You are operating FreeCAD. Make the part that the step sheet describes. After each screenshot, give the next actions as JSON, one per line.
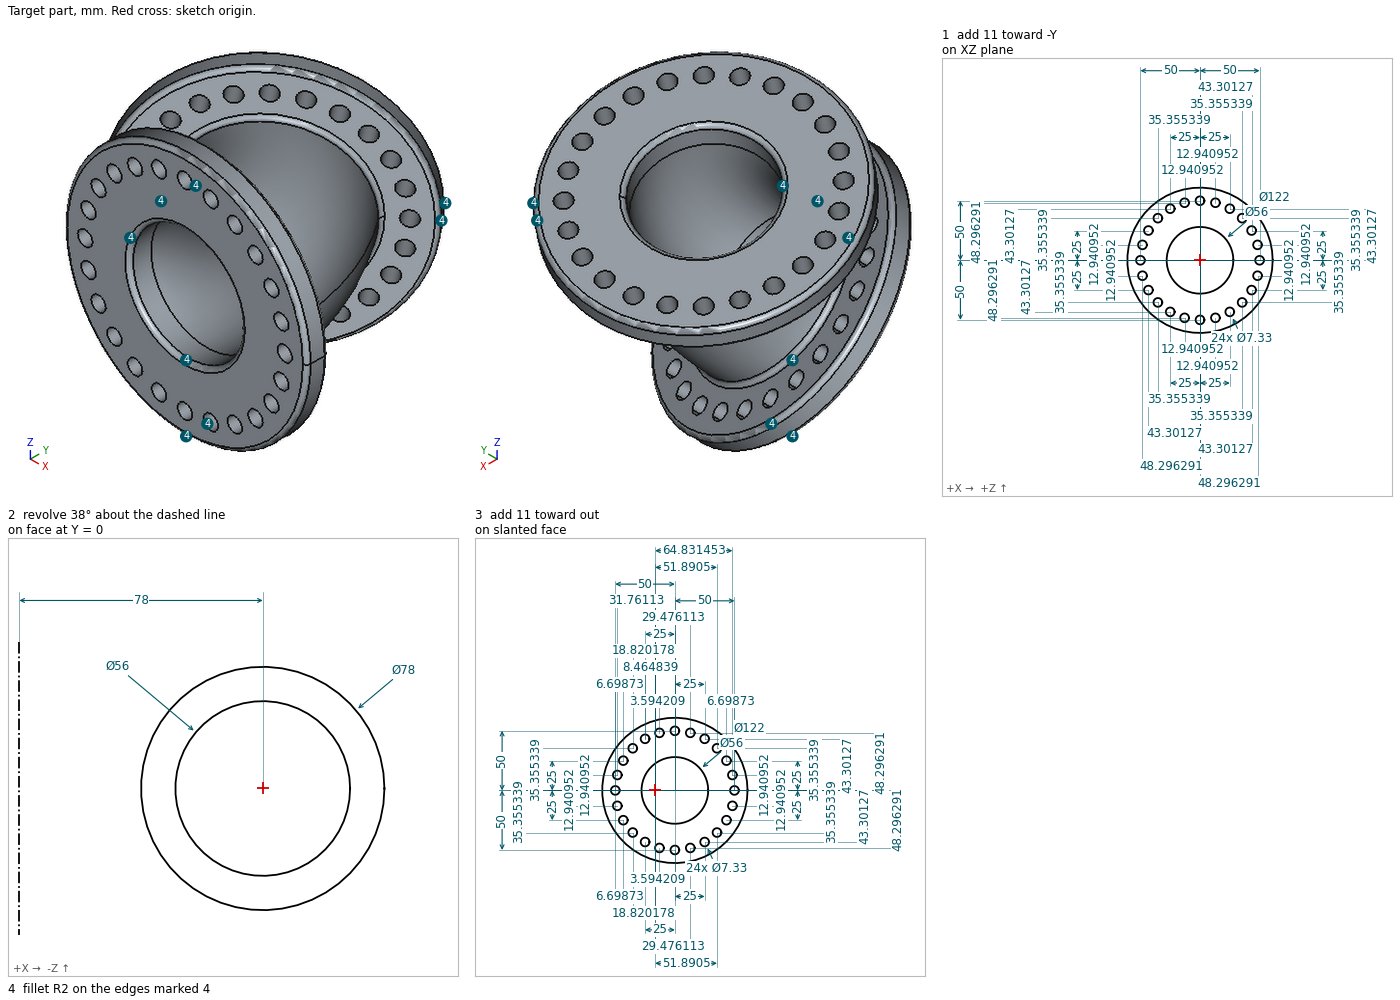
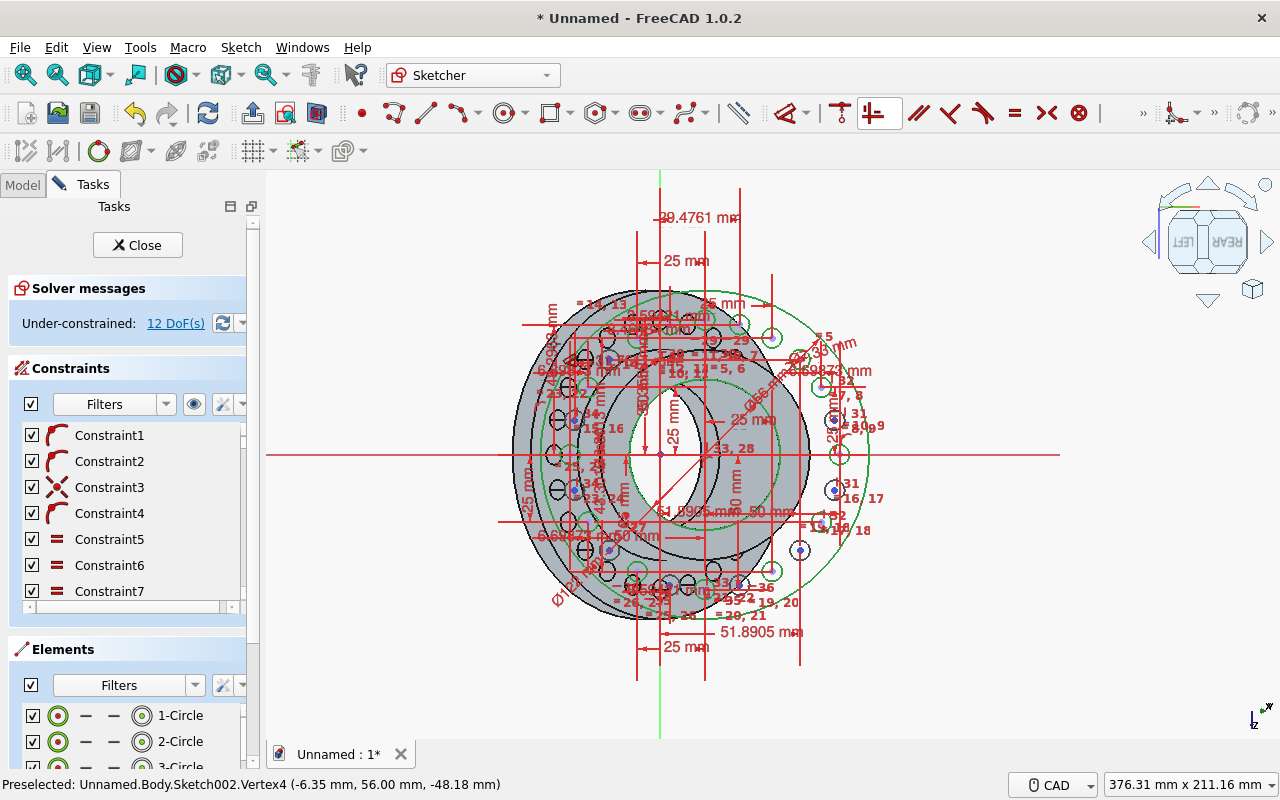
{"action": "left_click", "coordinate": [835, 420]}
{"action": "left_click", "coordinate": [809, 489]}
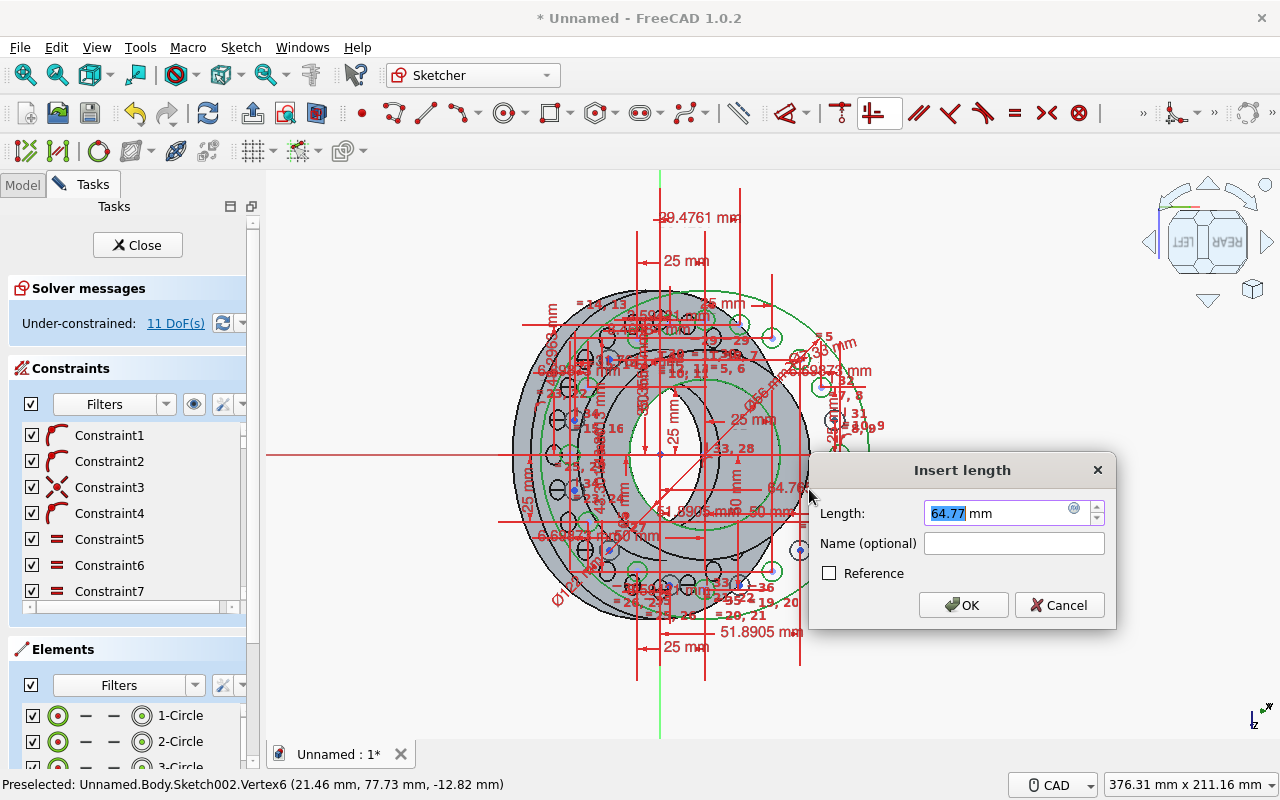
{"action": "type", "text": "64.831453"}
{"action": "key", "text": "Return"}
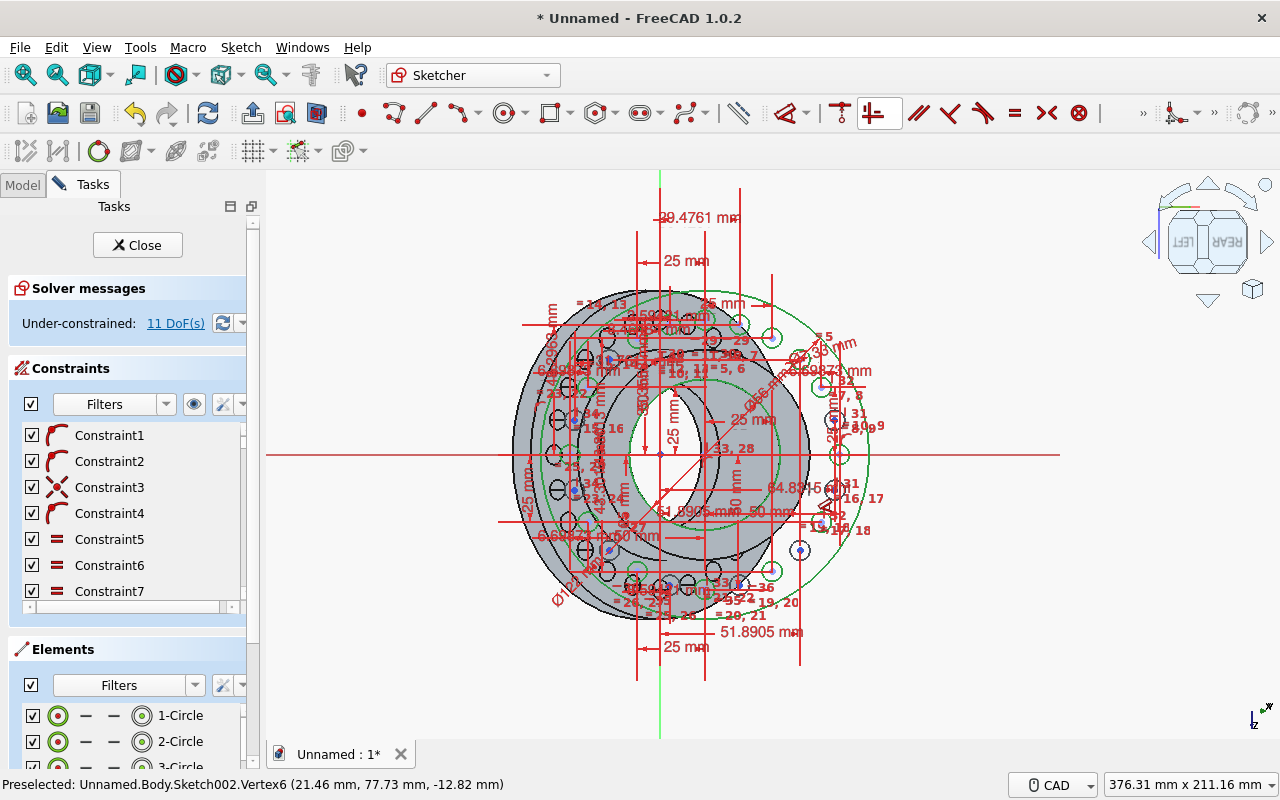
{"action": "left_click", "coordinate": [835, 420]}
{"action": "left_click", "coordinate": [917, 438]}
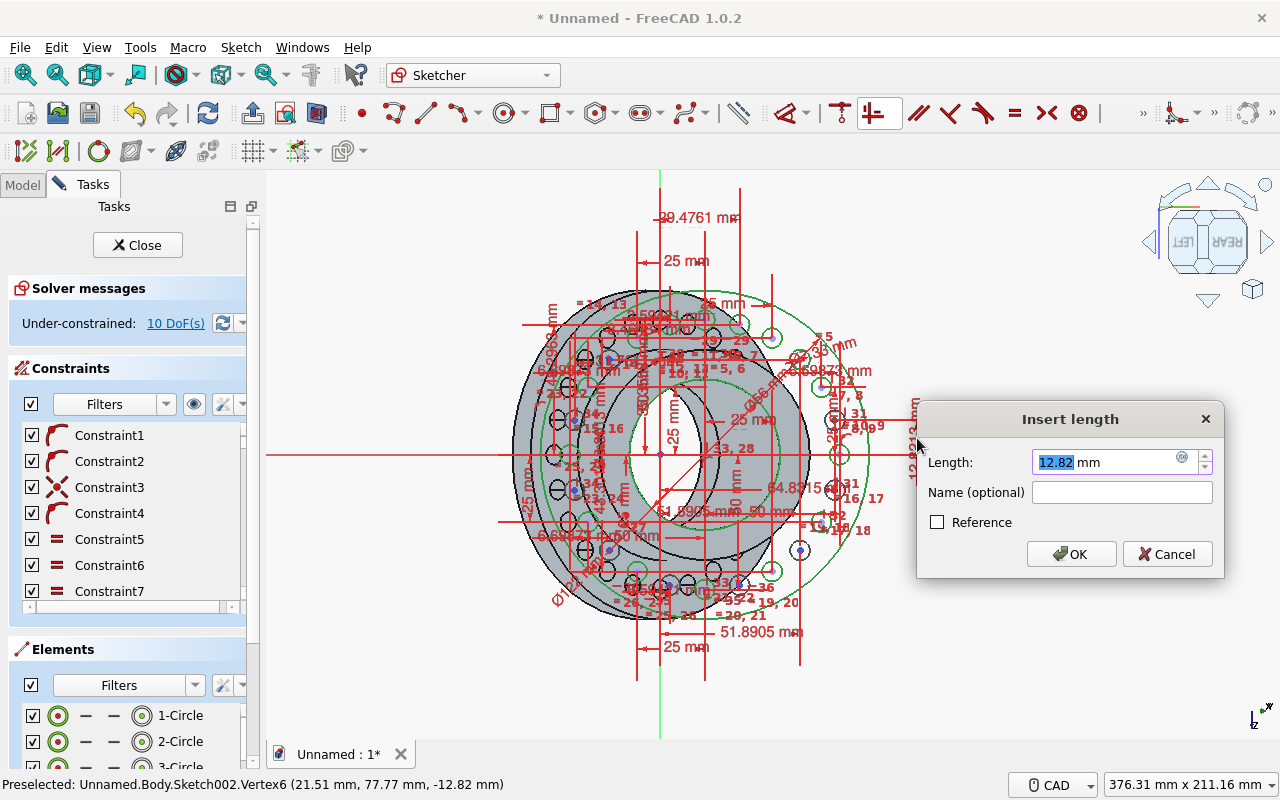
{"action": "type", "text": "12.940952"}
{"action": "key", "text": "Return"}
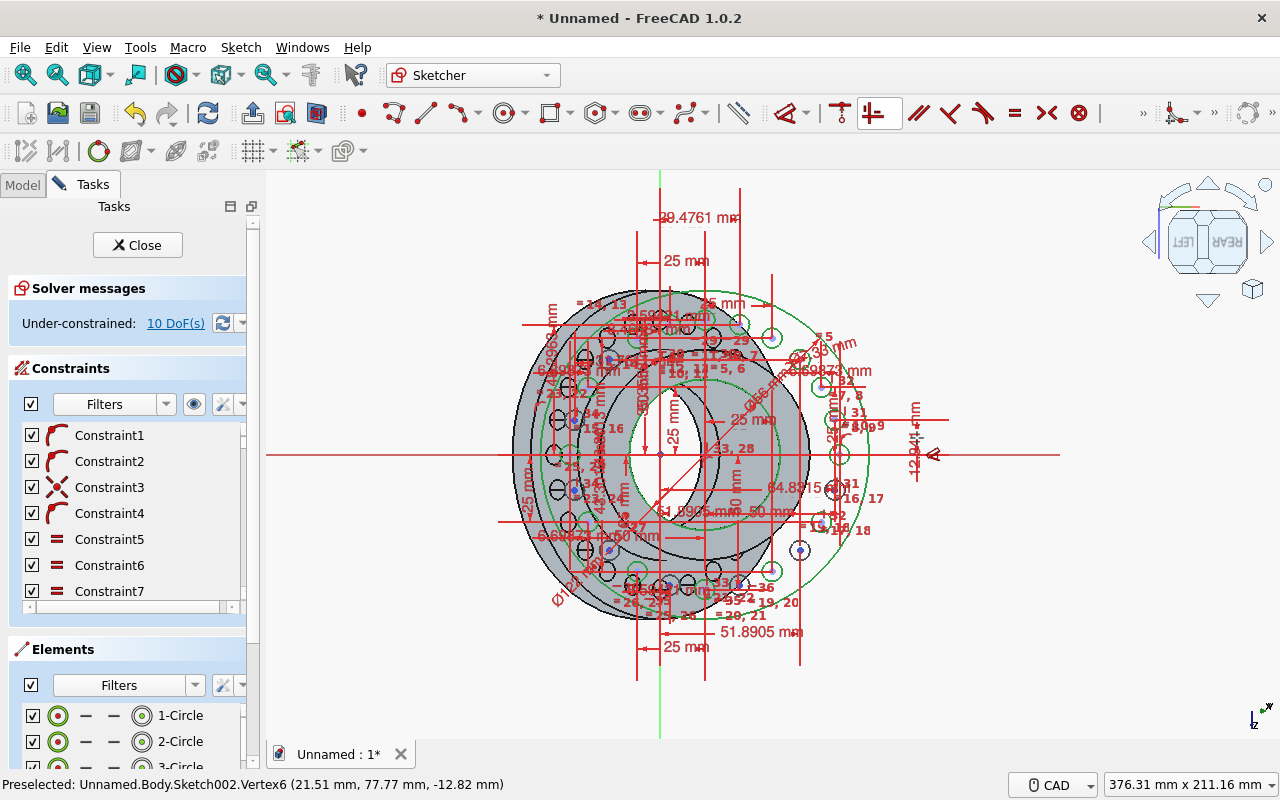
{"action": "left_click", "coordinate": [610, 360]}
{"action": "left_click", "coordinate": [623, 230]}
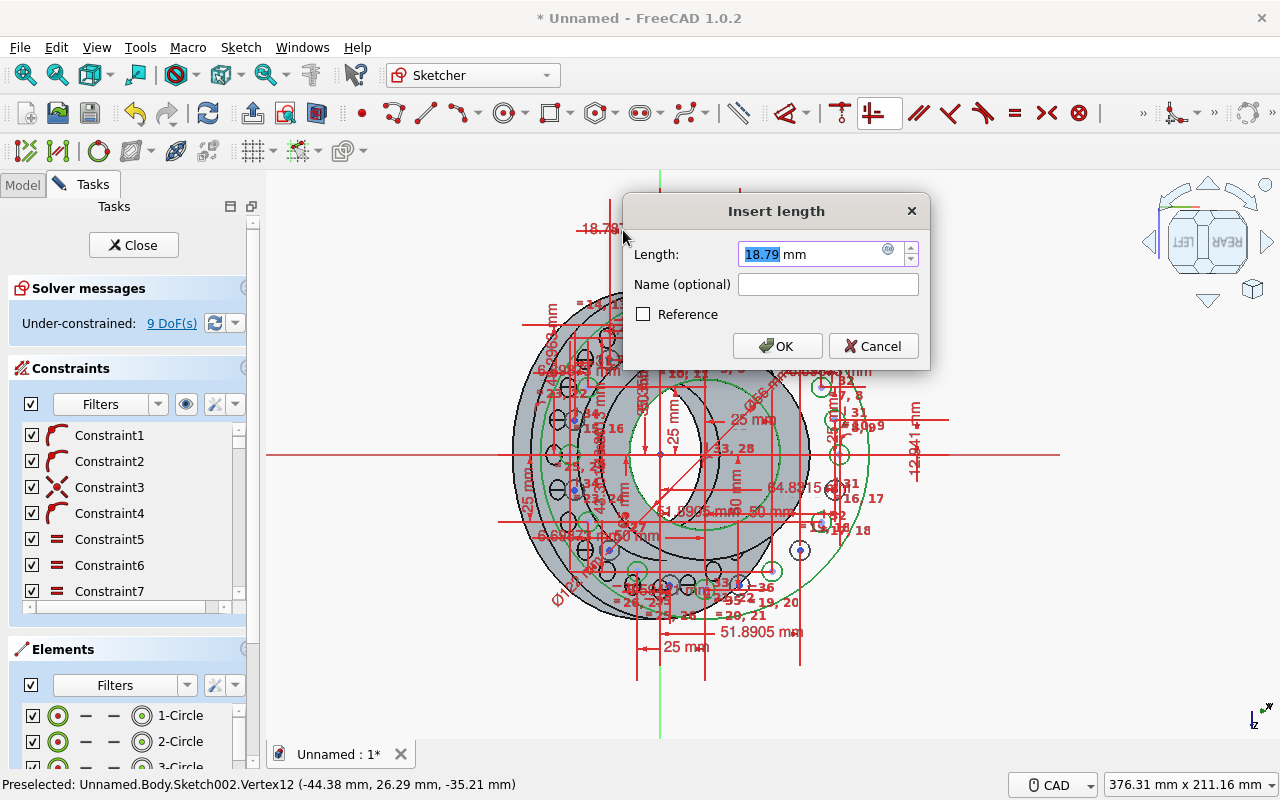
{"action": "type", "text": "18.820178"}
{"action": "key", "text": "Return"}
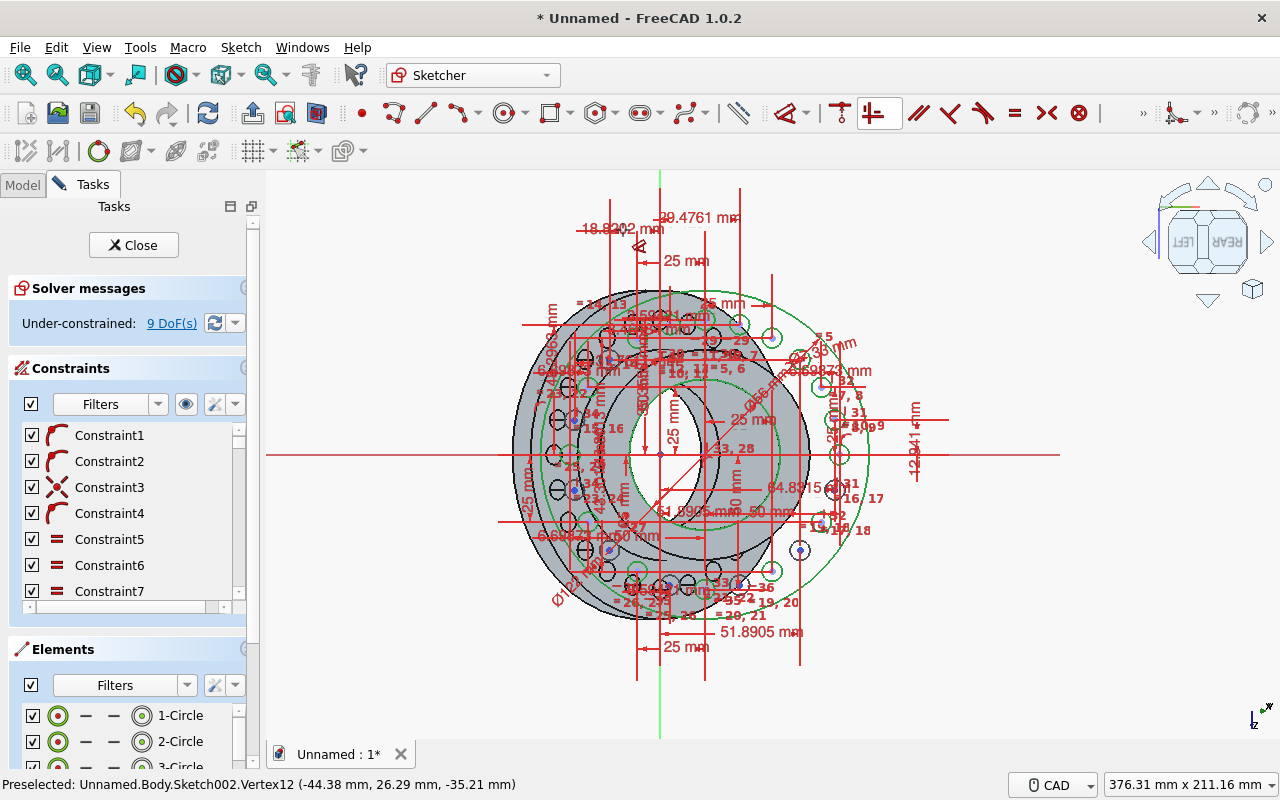
{"action": "left_click", "coordinate": [610, 360]}
{"action": "left_click", "coordinate": [528, 407]}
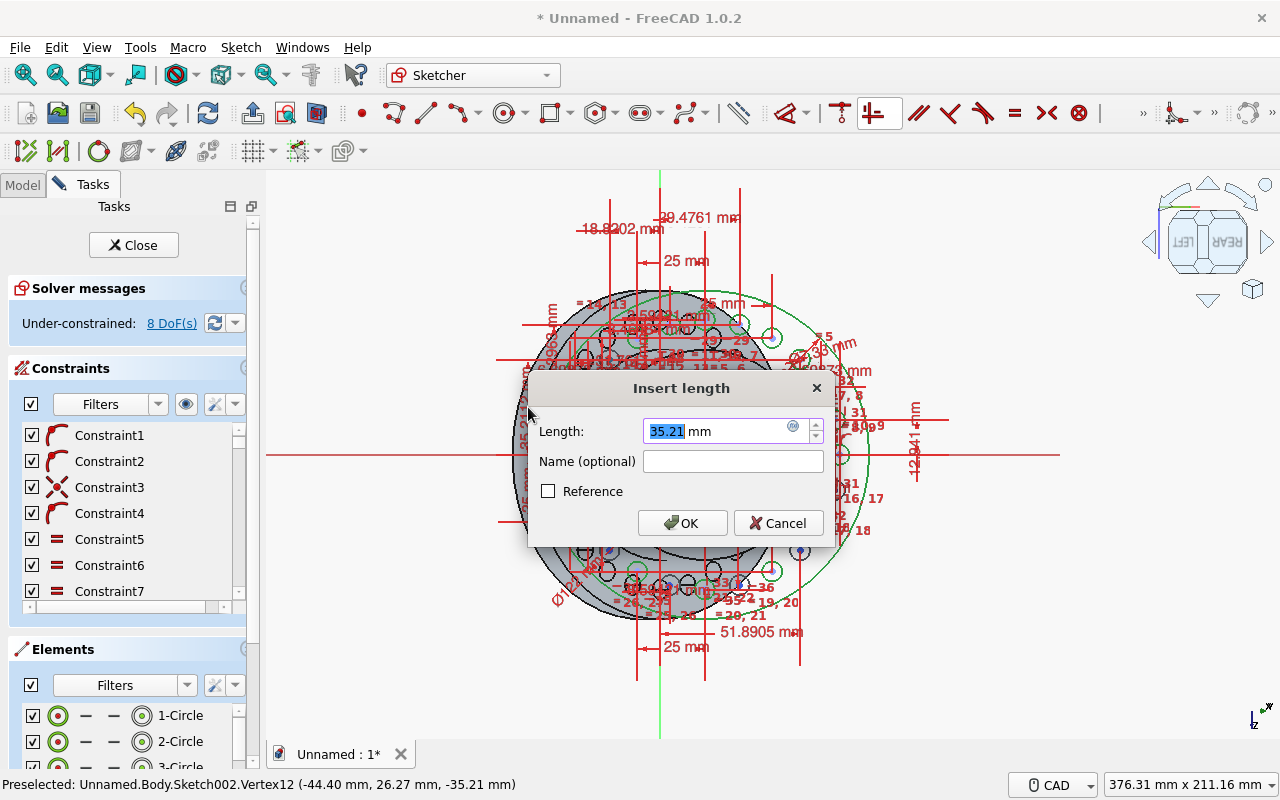
{"action": "type", "text": "35.355339"}
{"action": "key", "text": "Return"}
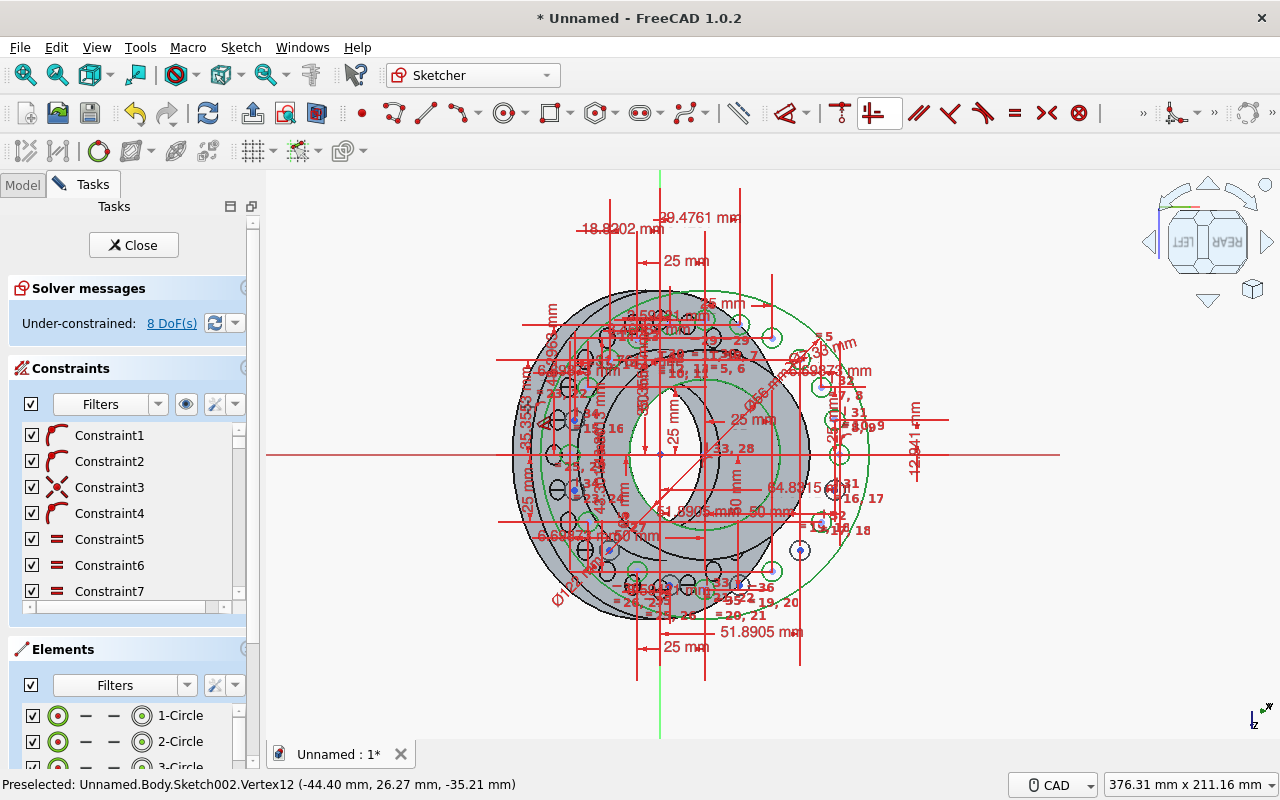
{"action": "left_click", "coordinate": [575, 420]}
{"action": "left_click", "coordinate": [517, 438]}